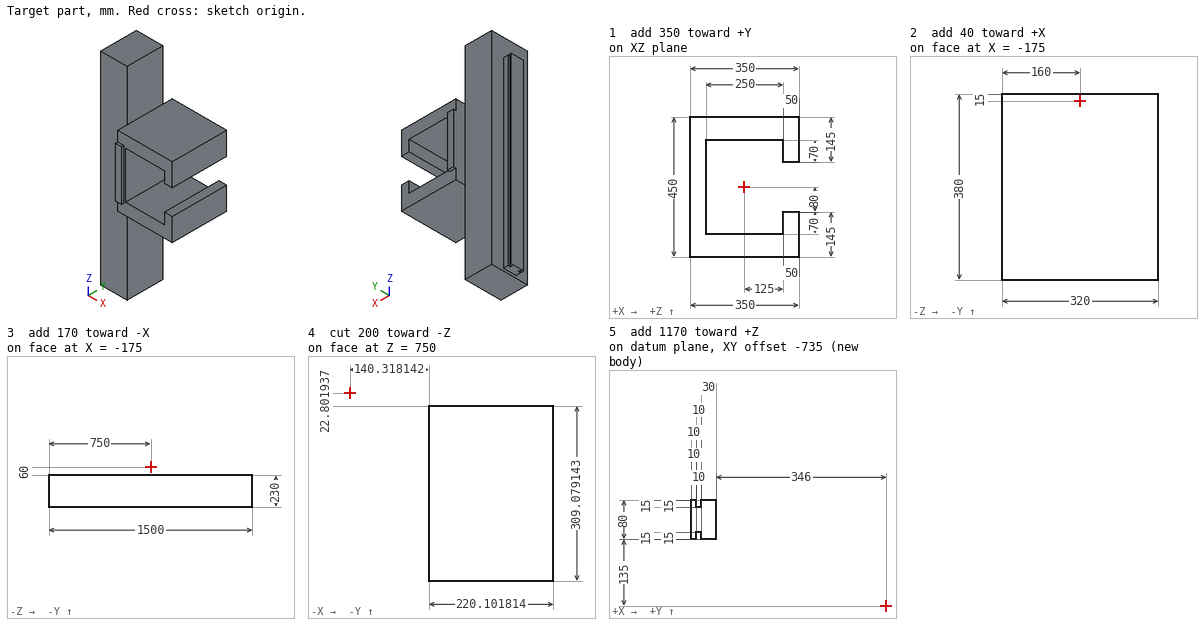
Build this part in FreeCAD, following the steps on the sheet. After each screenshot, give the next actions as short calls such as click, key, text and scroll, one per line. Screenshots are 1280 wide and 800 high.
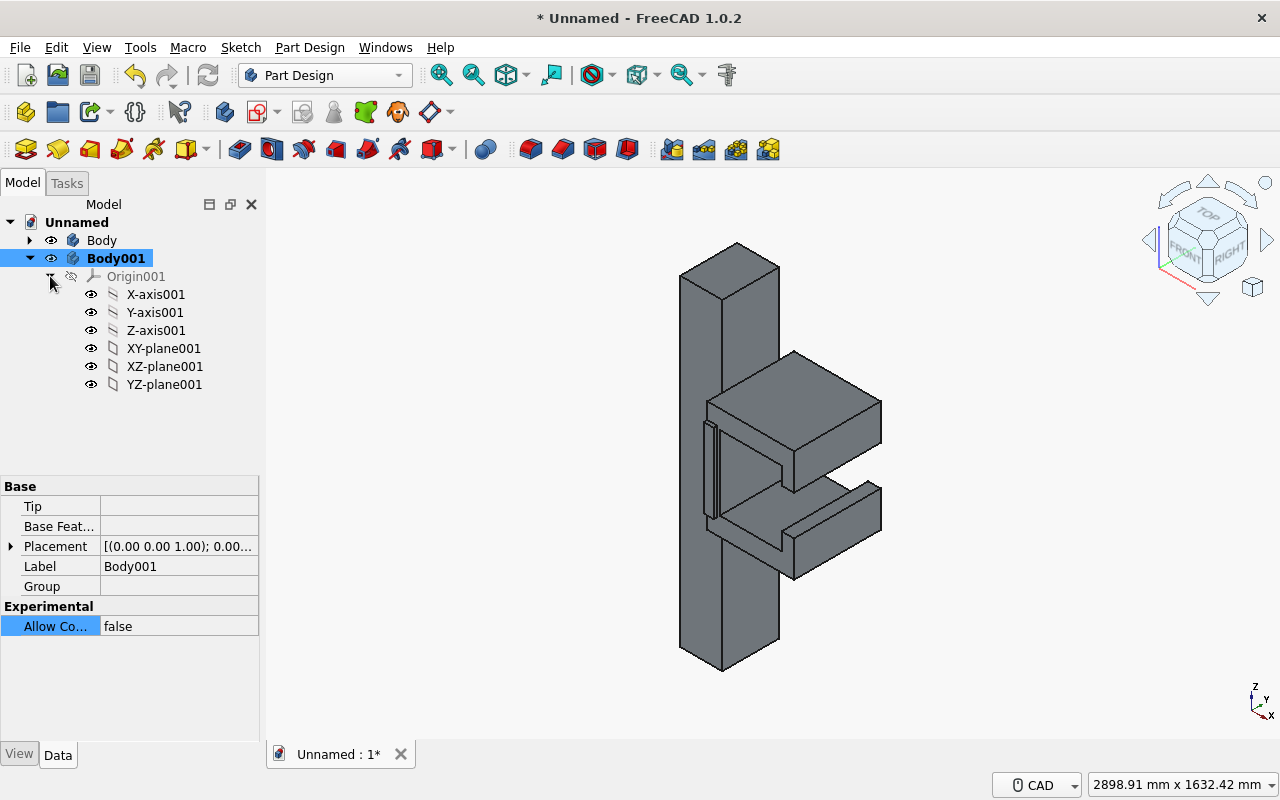
click(136, 348)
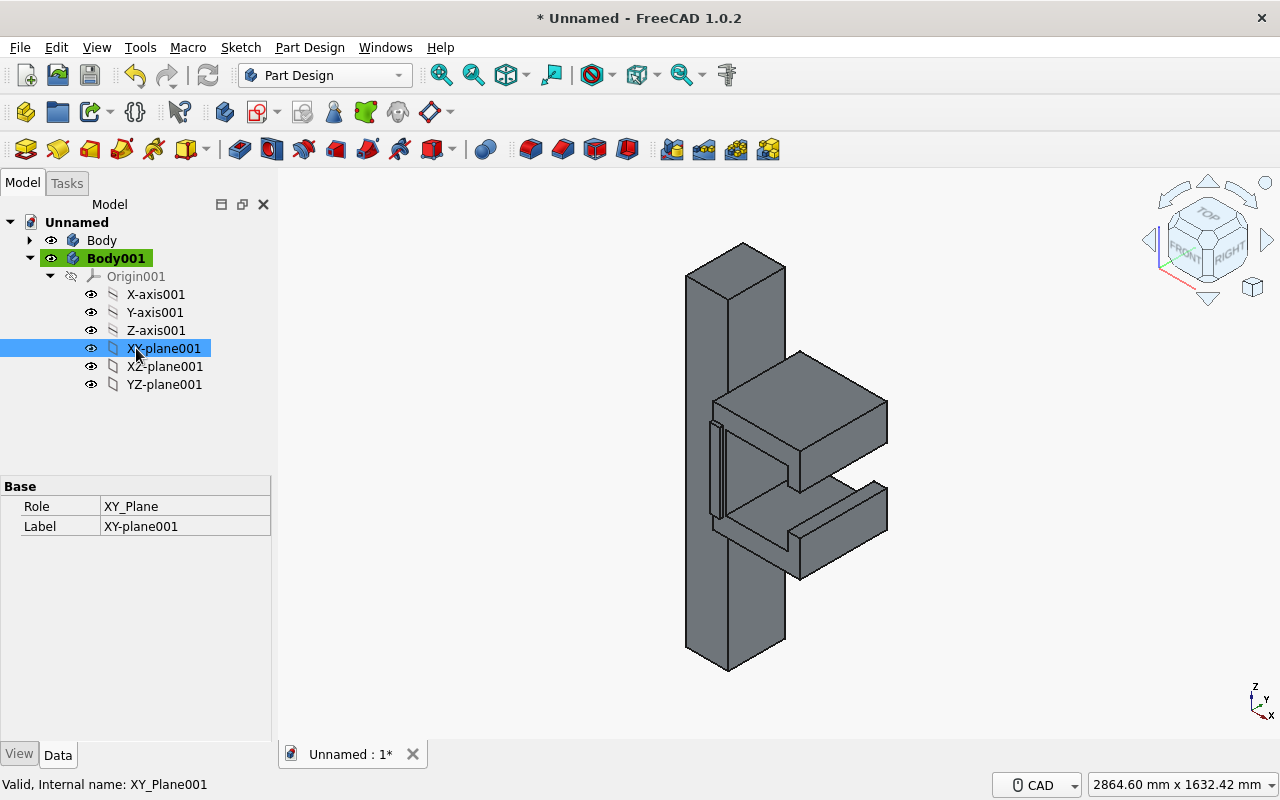
click(430, 112)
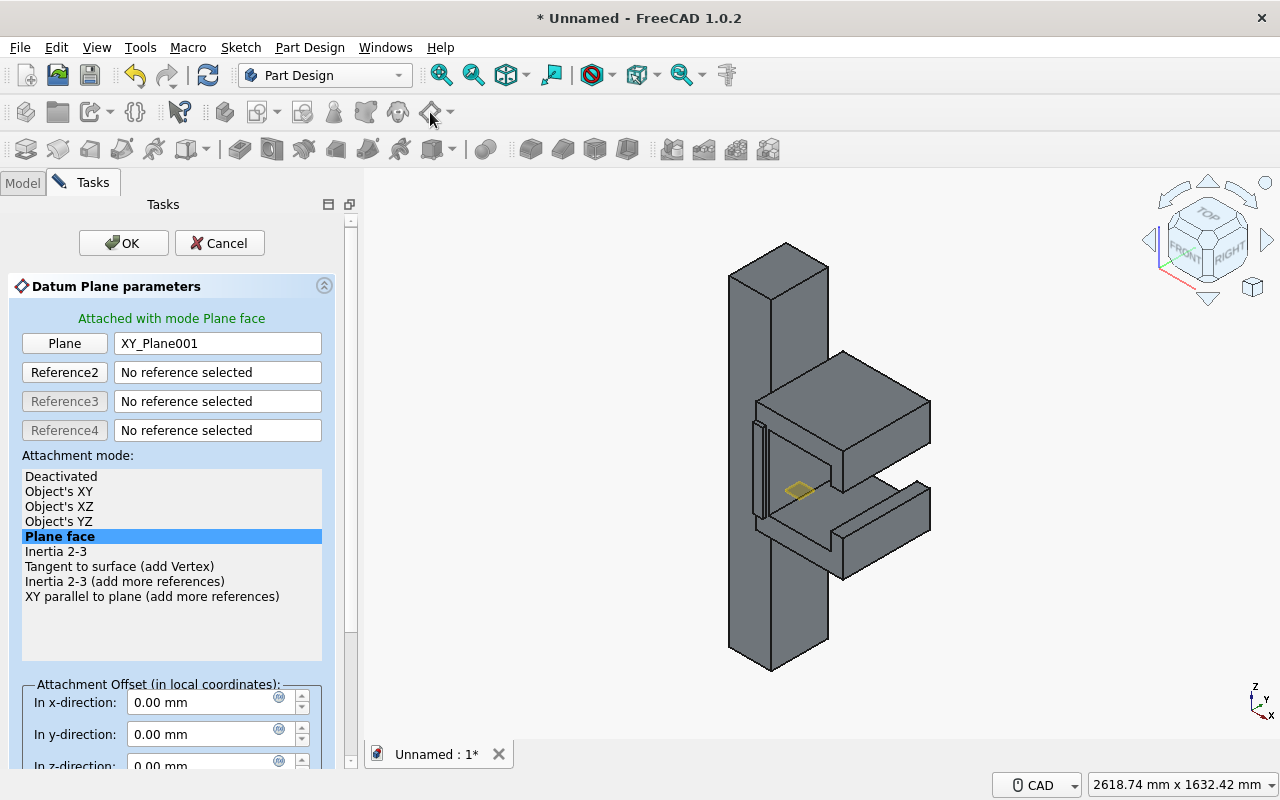
scroll(351, 491, down, 2)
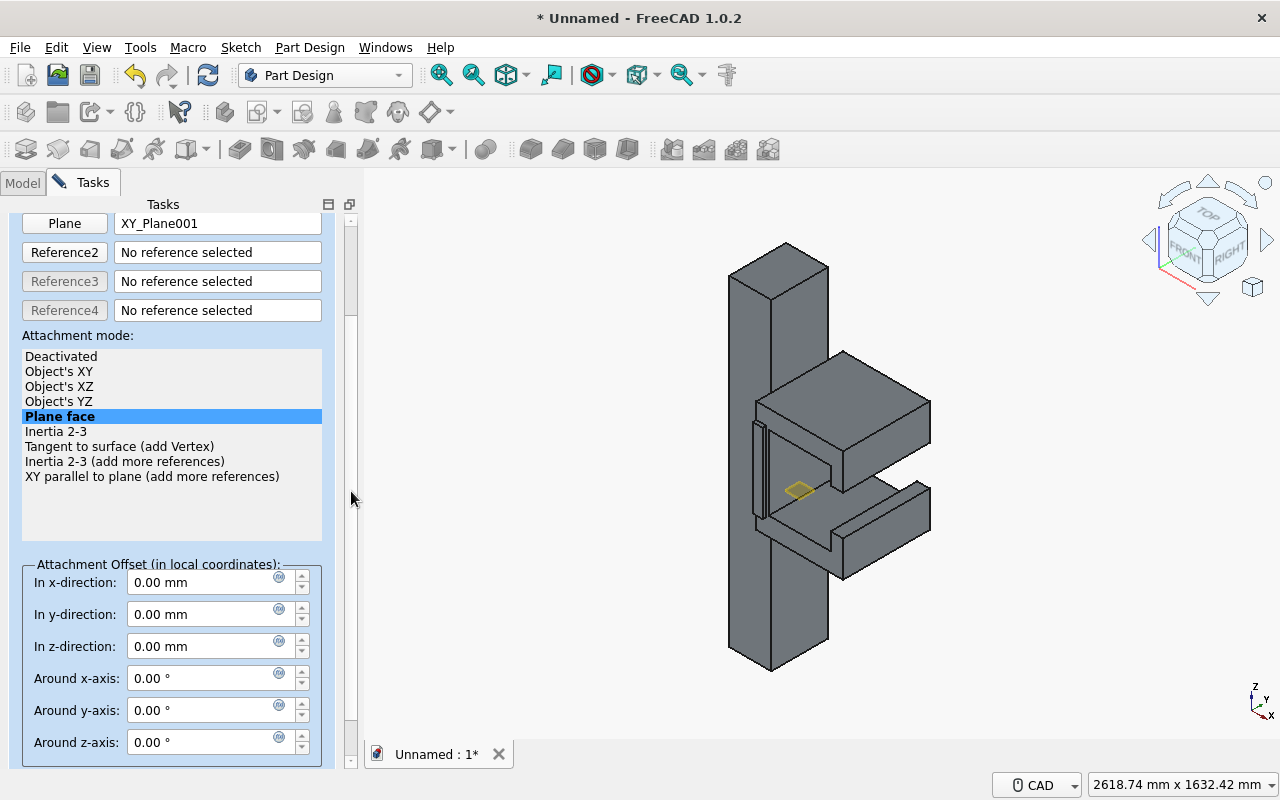
triple_click(210, 646)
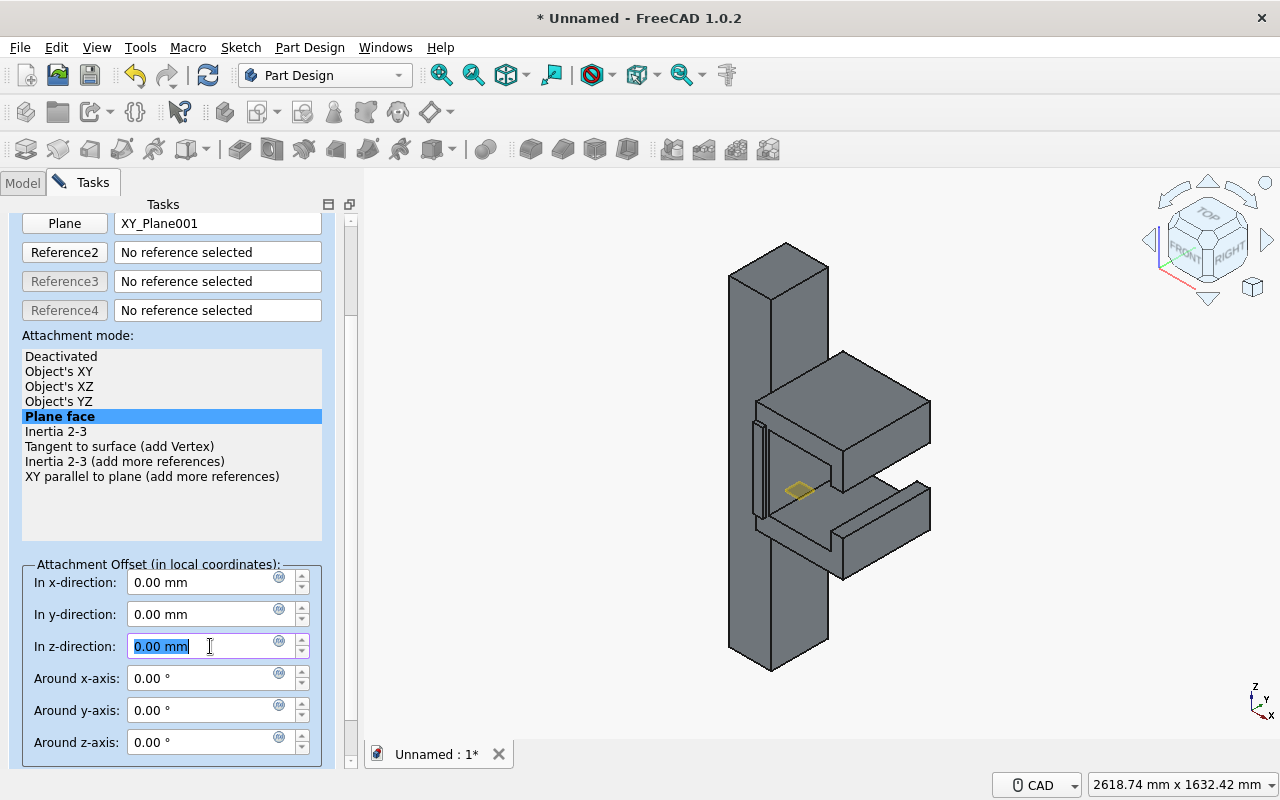
text(-735)
key(Tab)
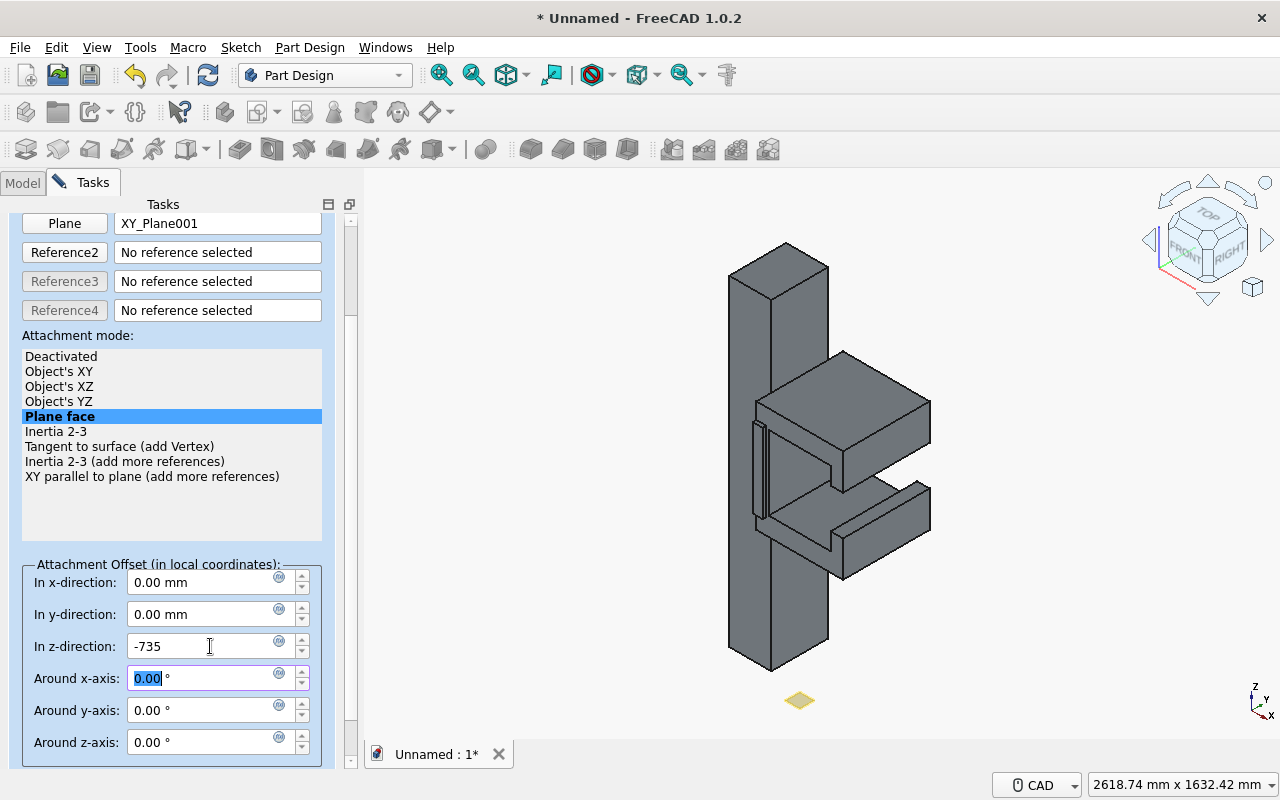
scroll(351, 491, up, 3)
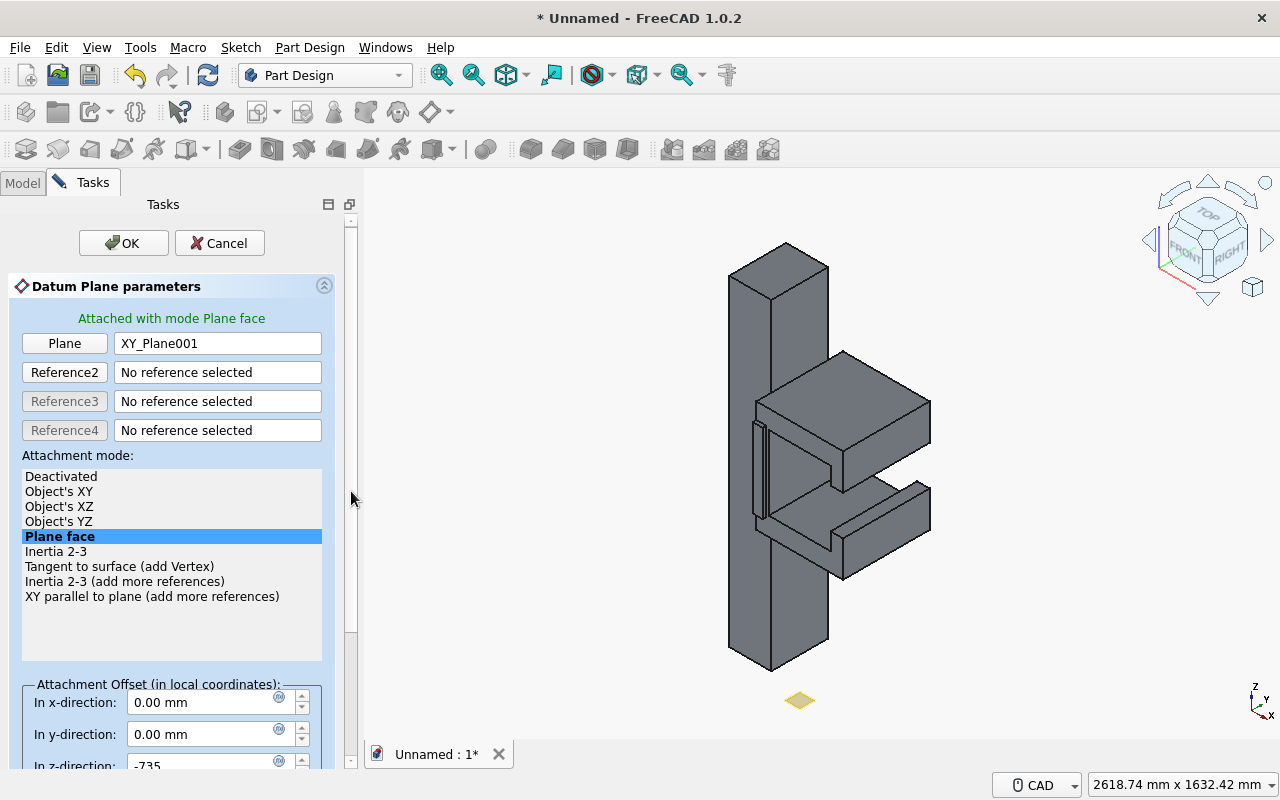
click(124, 243)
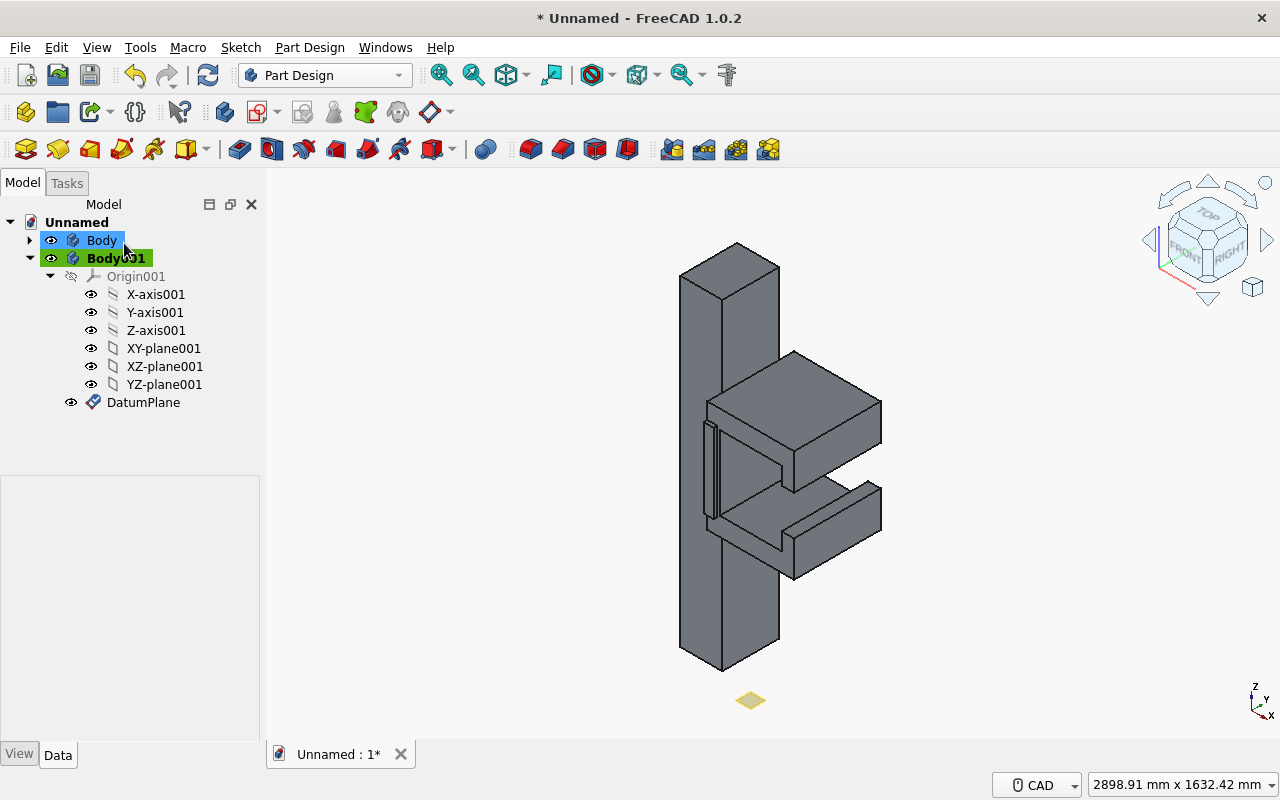
click(116, 402)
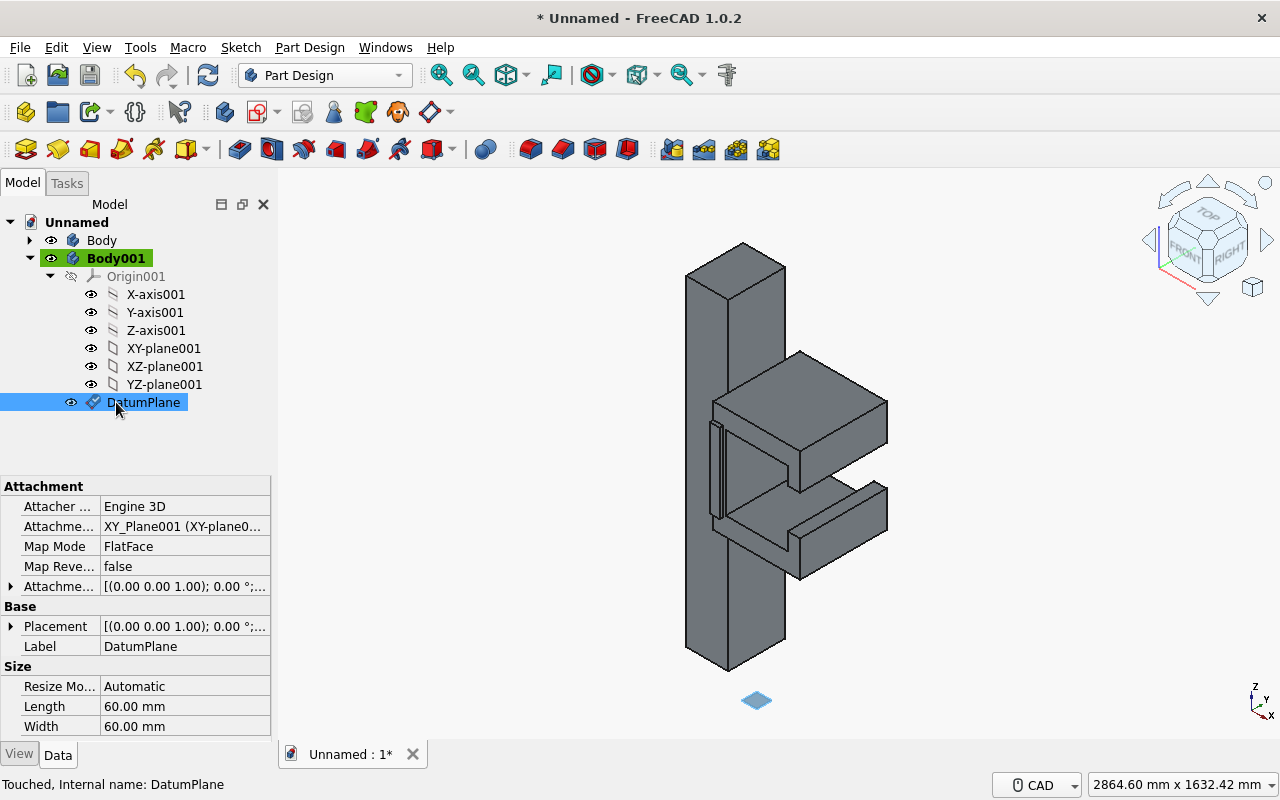
click(258, 112)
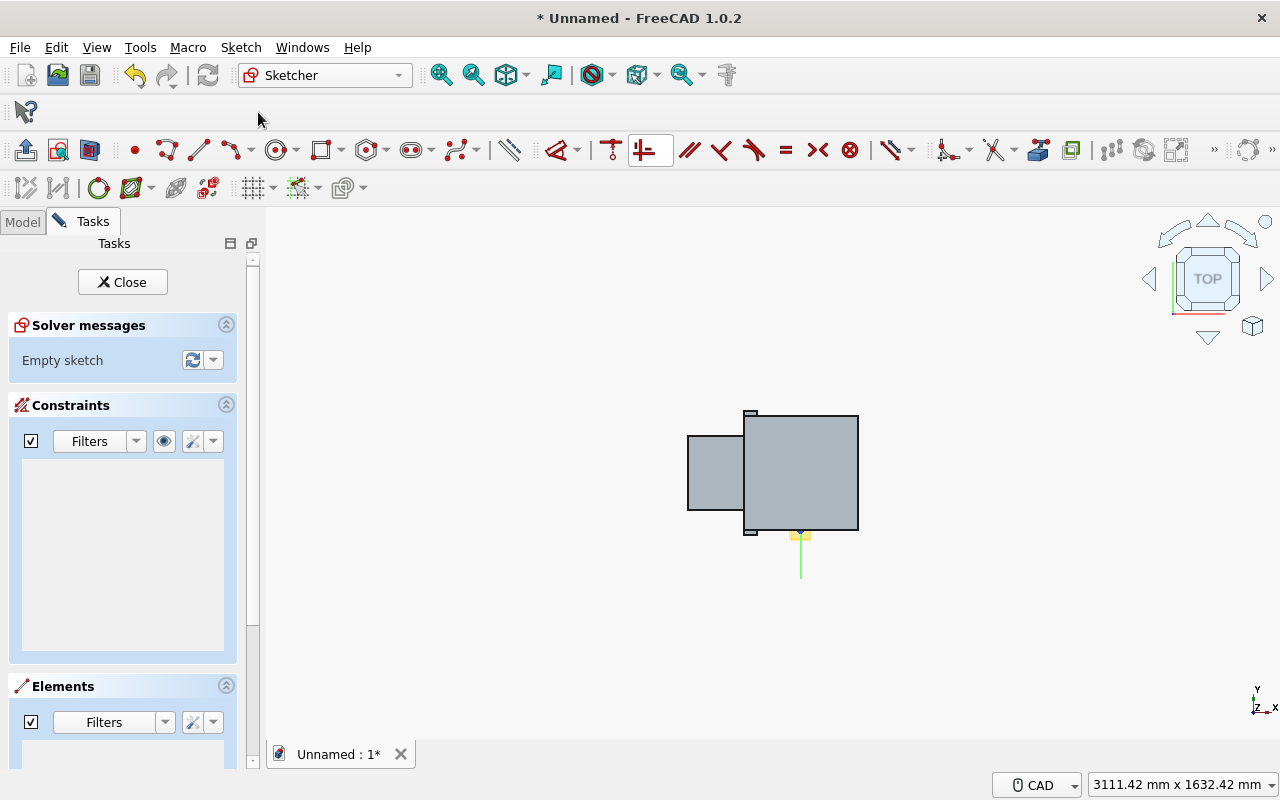
scroll(678, 473, up, 13)